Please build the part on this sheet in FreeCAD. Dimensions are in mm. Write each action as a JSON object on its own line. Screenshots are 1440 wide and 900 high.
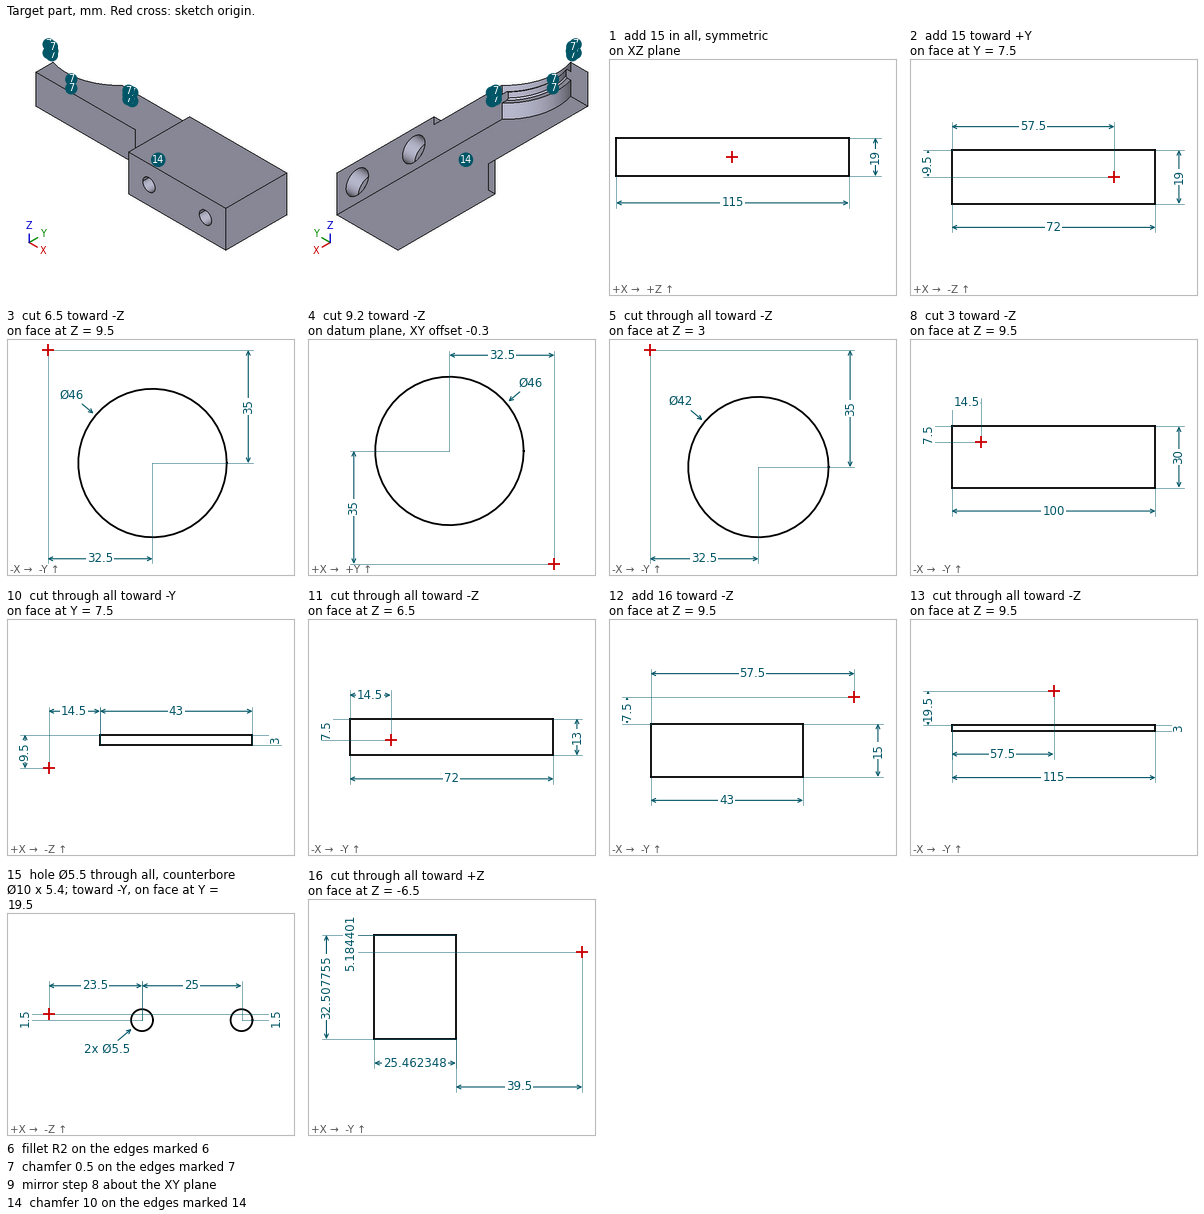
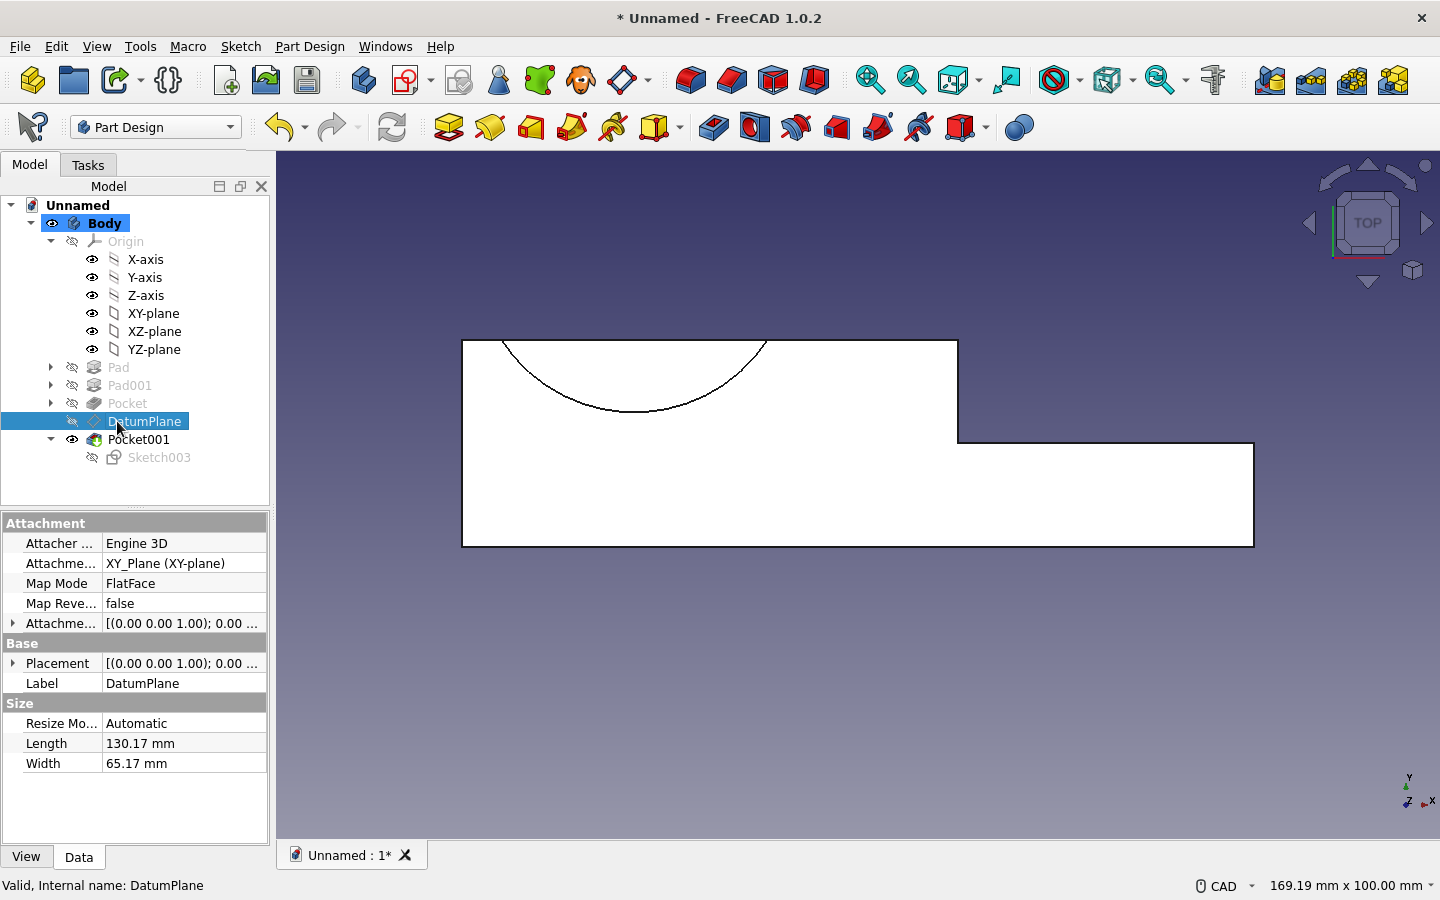
{"action": "left_click", "coordinate": [634, 375]}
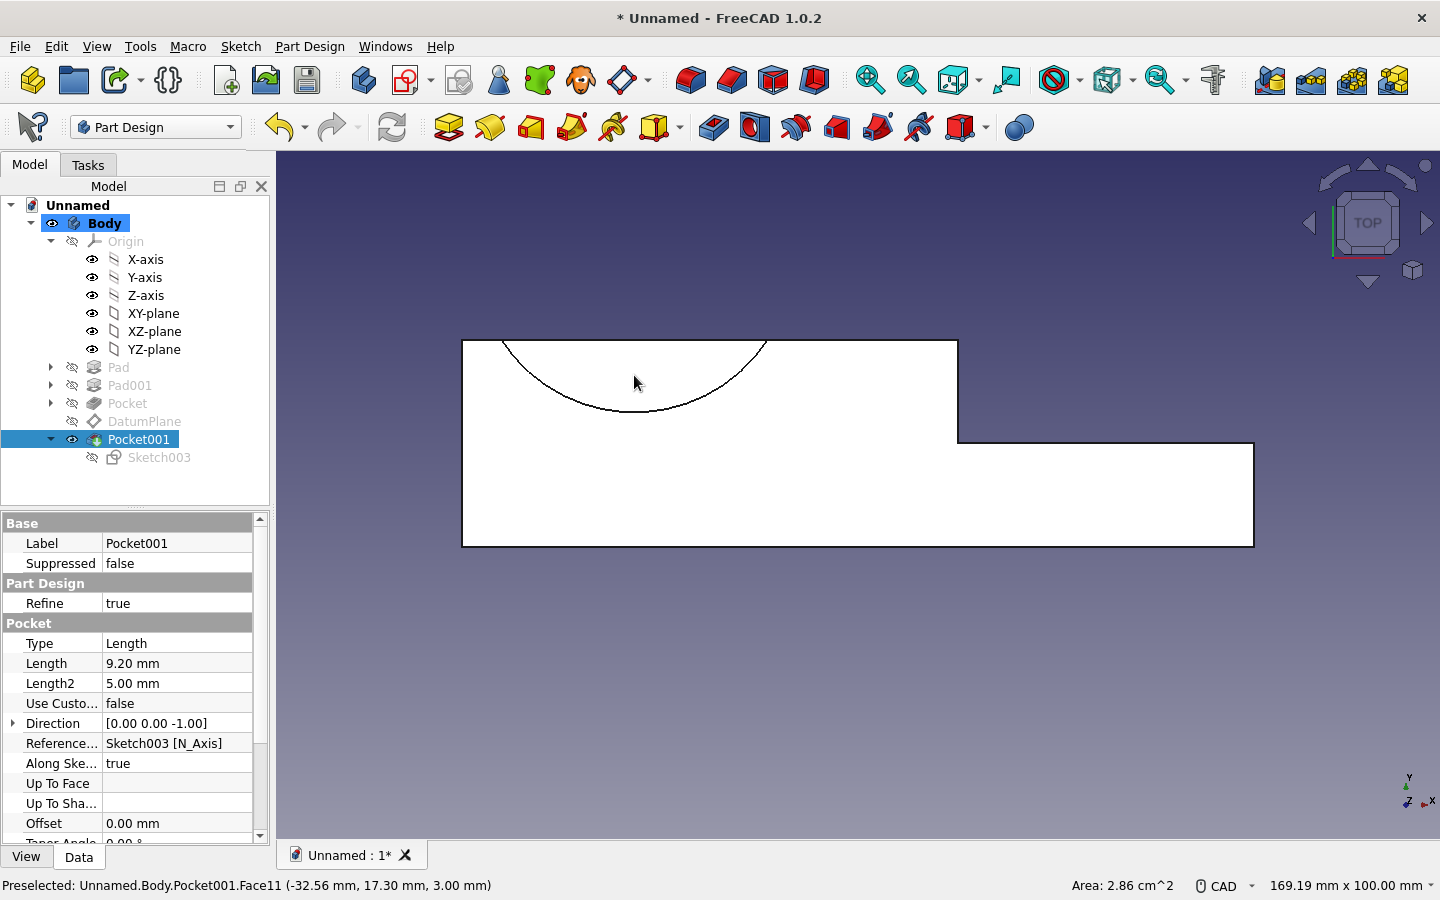
{"action": "left_click", "coordinate": [404, 80]}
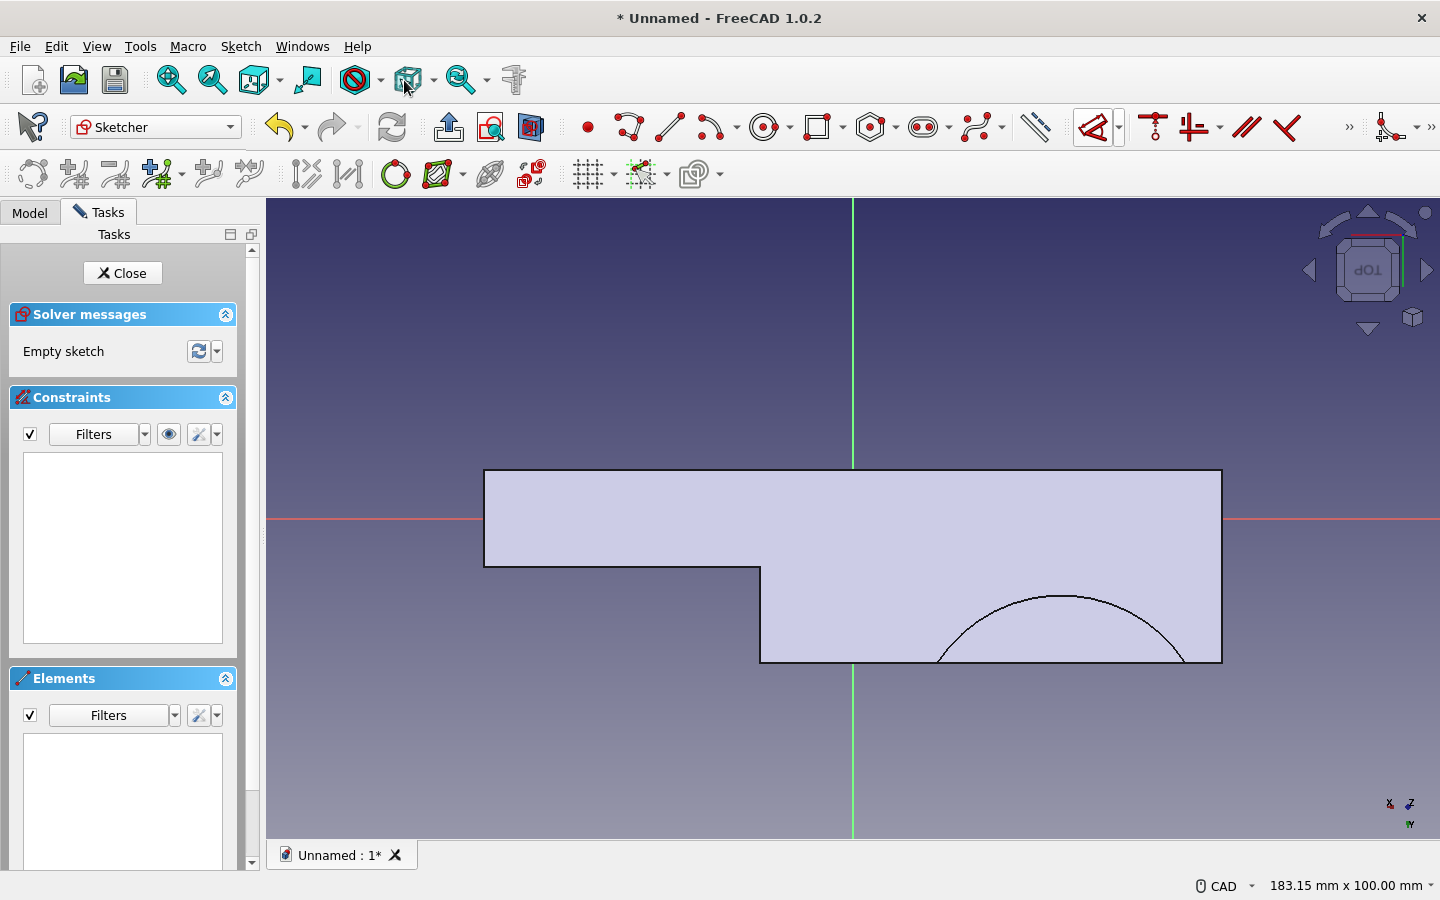
{"action": "scroll", "coordinate": [294, 226], "scroll_direction": "down", "scroll_amount": 1}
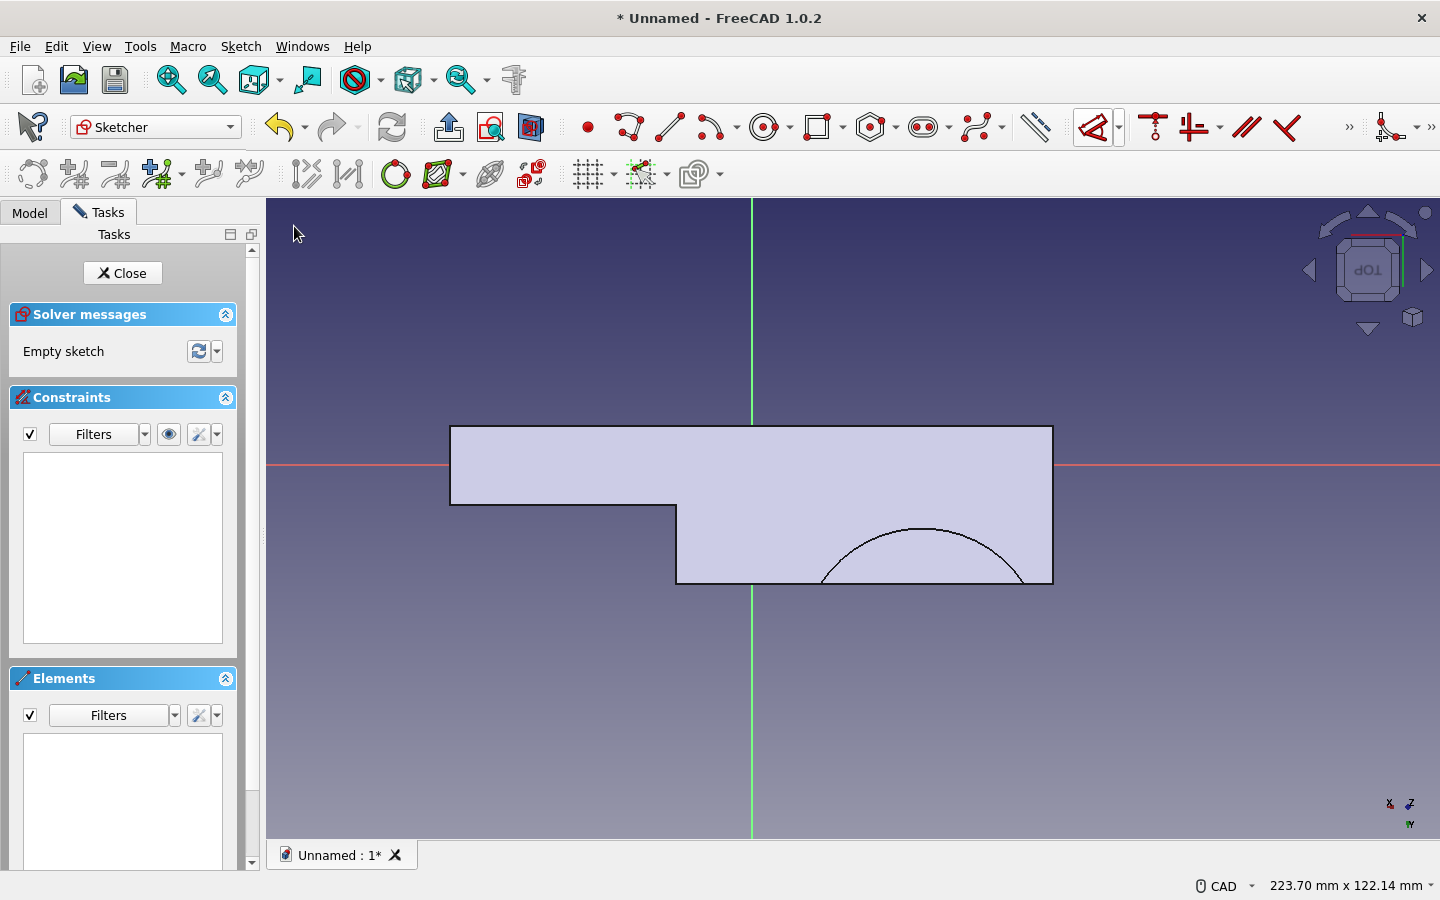
{"action": "scroll", "coordinate": [1111, 803], "scroll_direction": "up", "scroll_amount": 2}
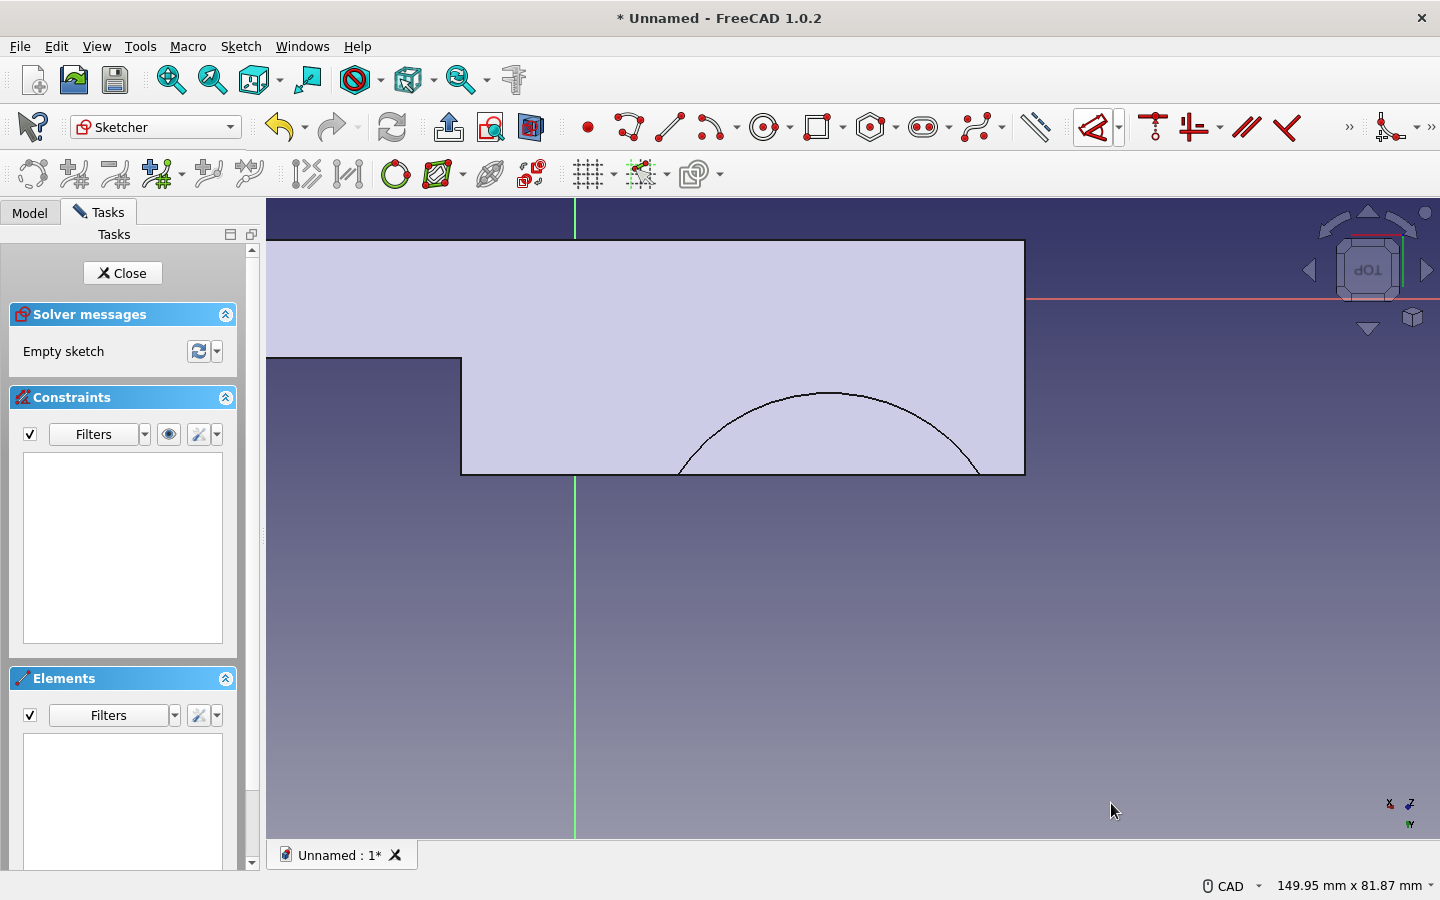
{"action": "left_click", "coordinate": [764, 128]}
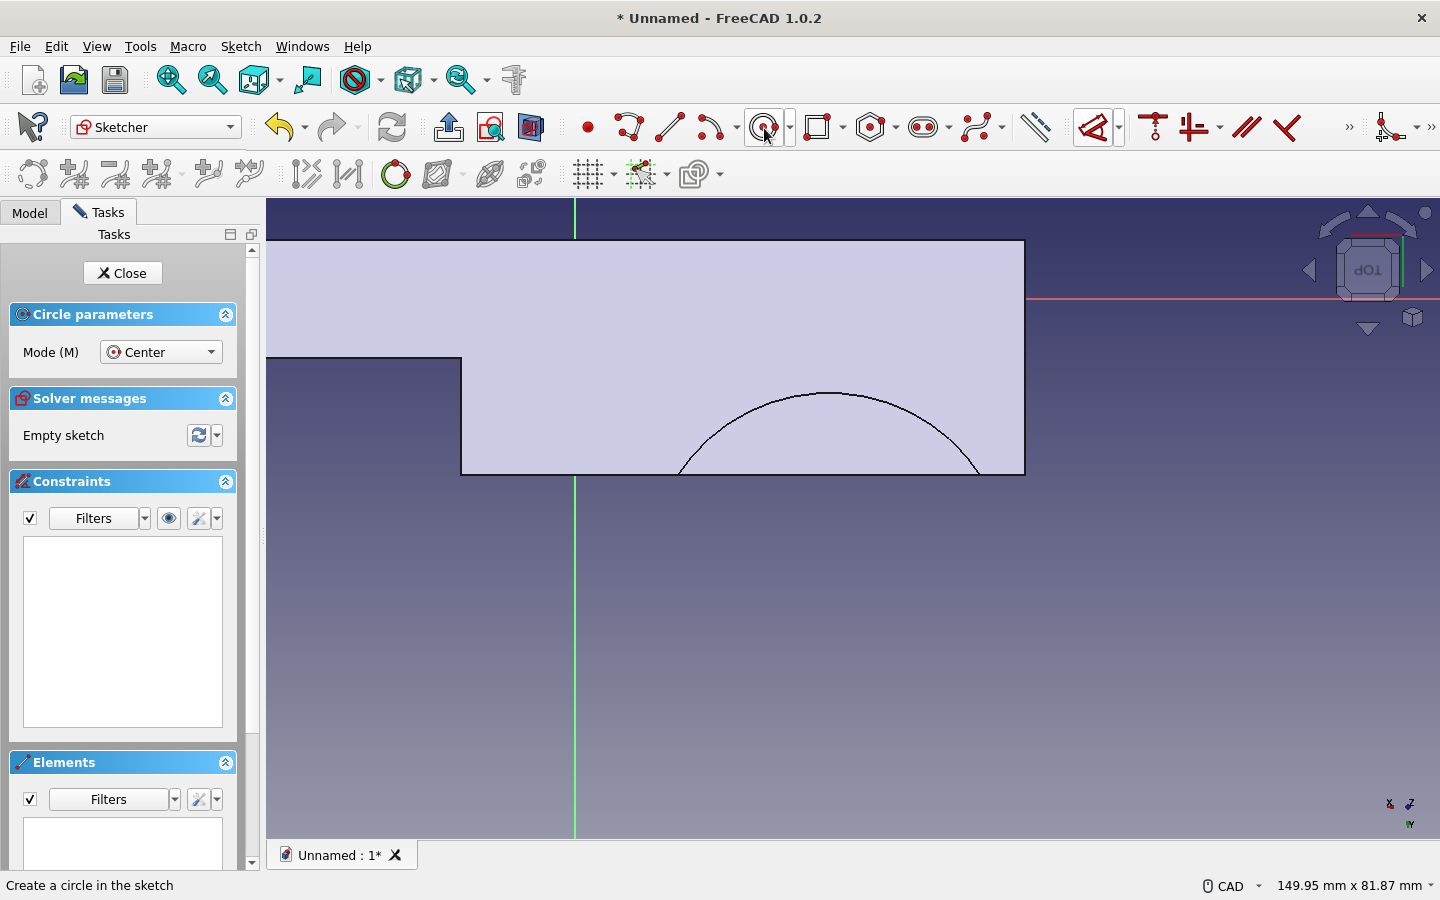
{"action": "left_click", "coordinate": [829, 573]}
{"action": "mouse_move", "coordinate": [945, 457]}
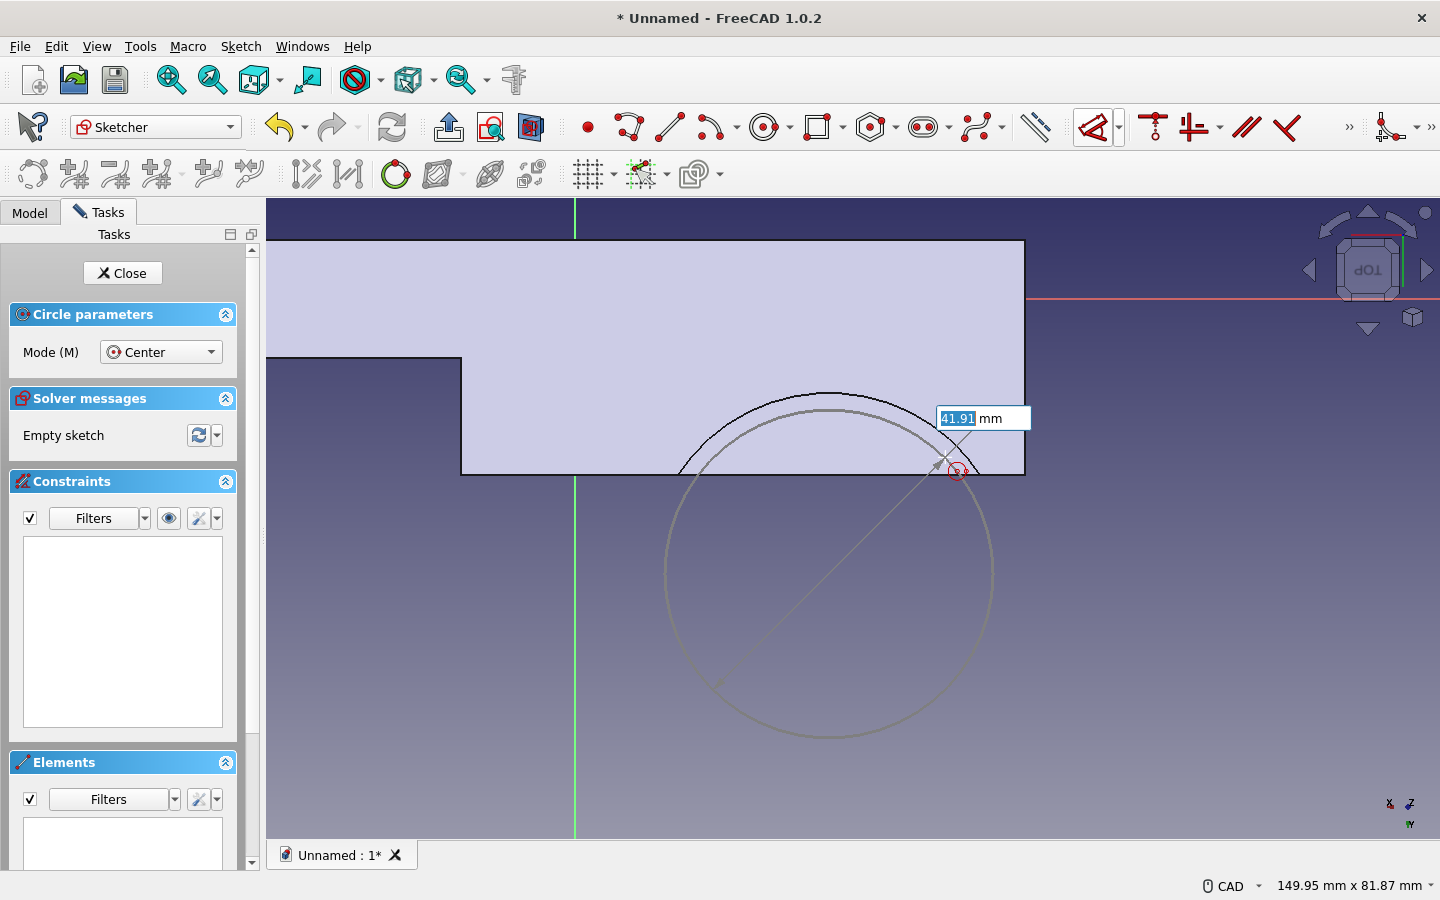
{"action": "type", "text": "42"}
{"action": "key", "text": "Return"}
{"action": "key", "text": "Escape"}